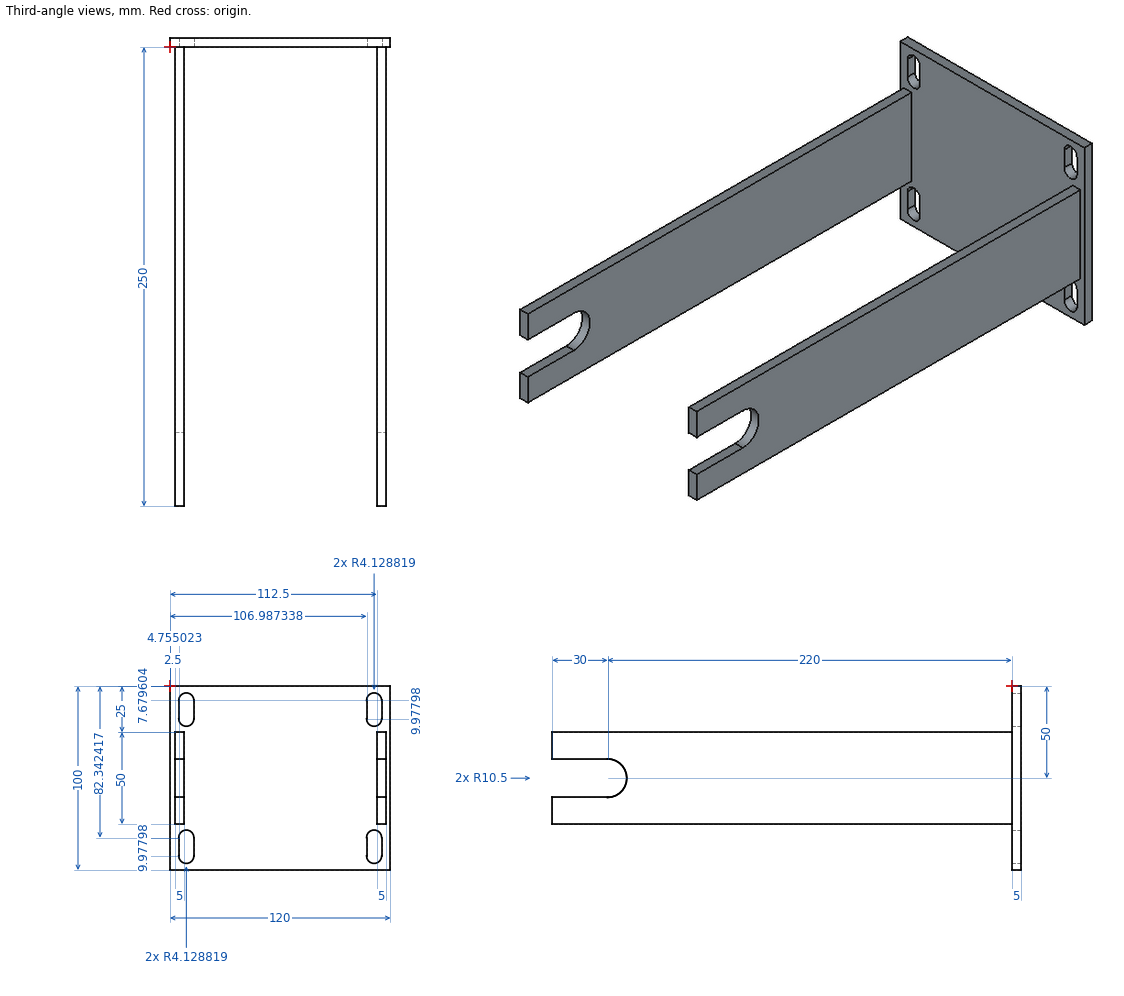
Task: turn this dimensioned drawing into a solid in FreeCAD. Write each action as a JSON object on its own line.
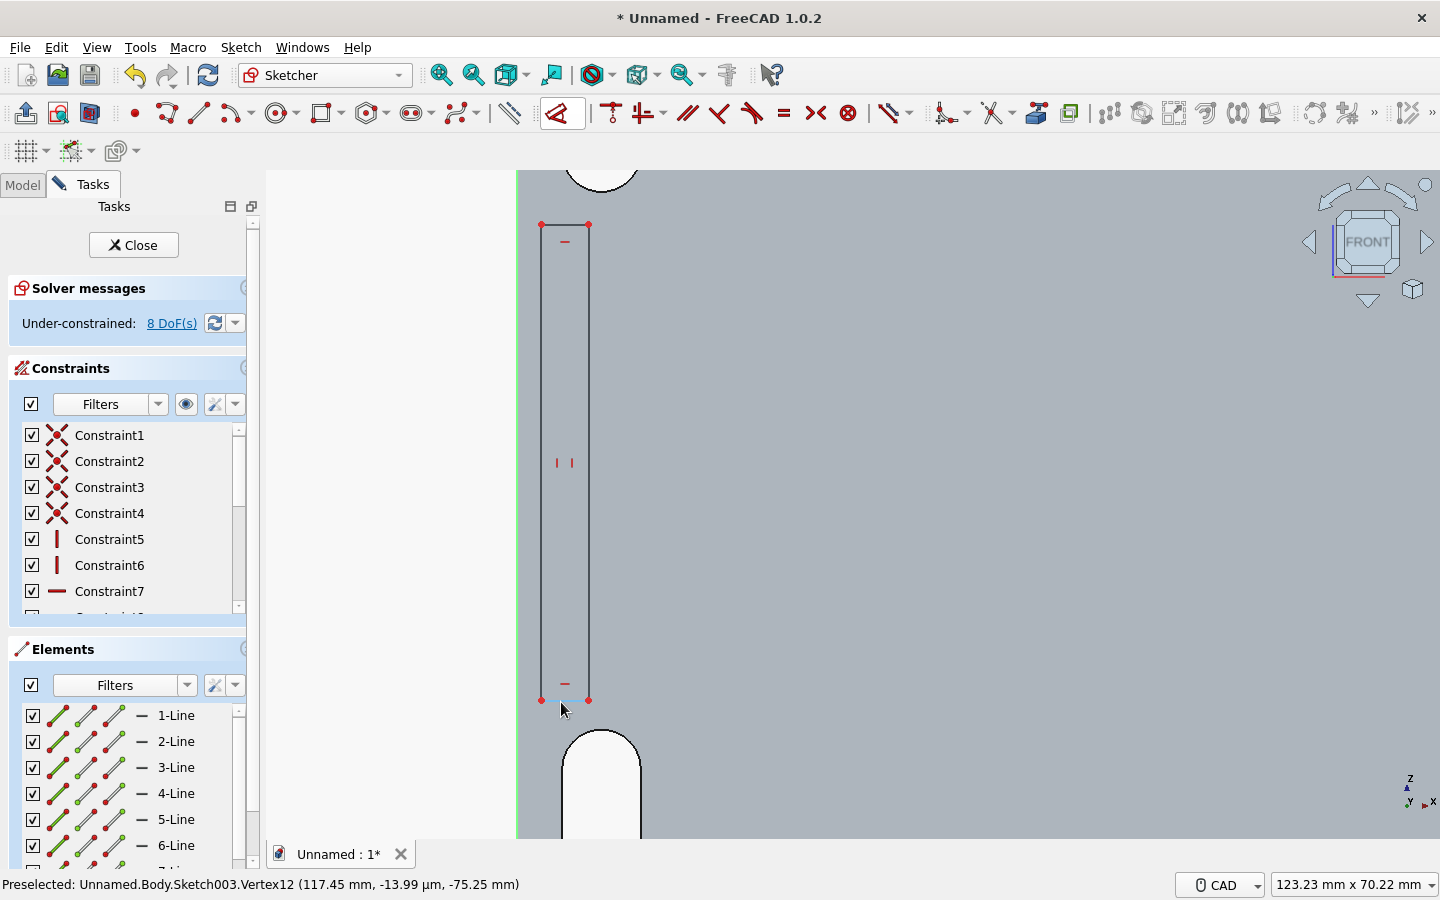
{"action": "left_click", "coordinate": [560, 701]}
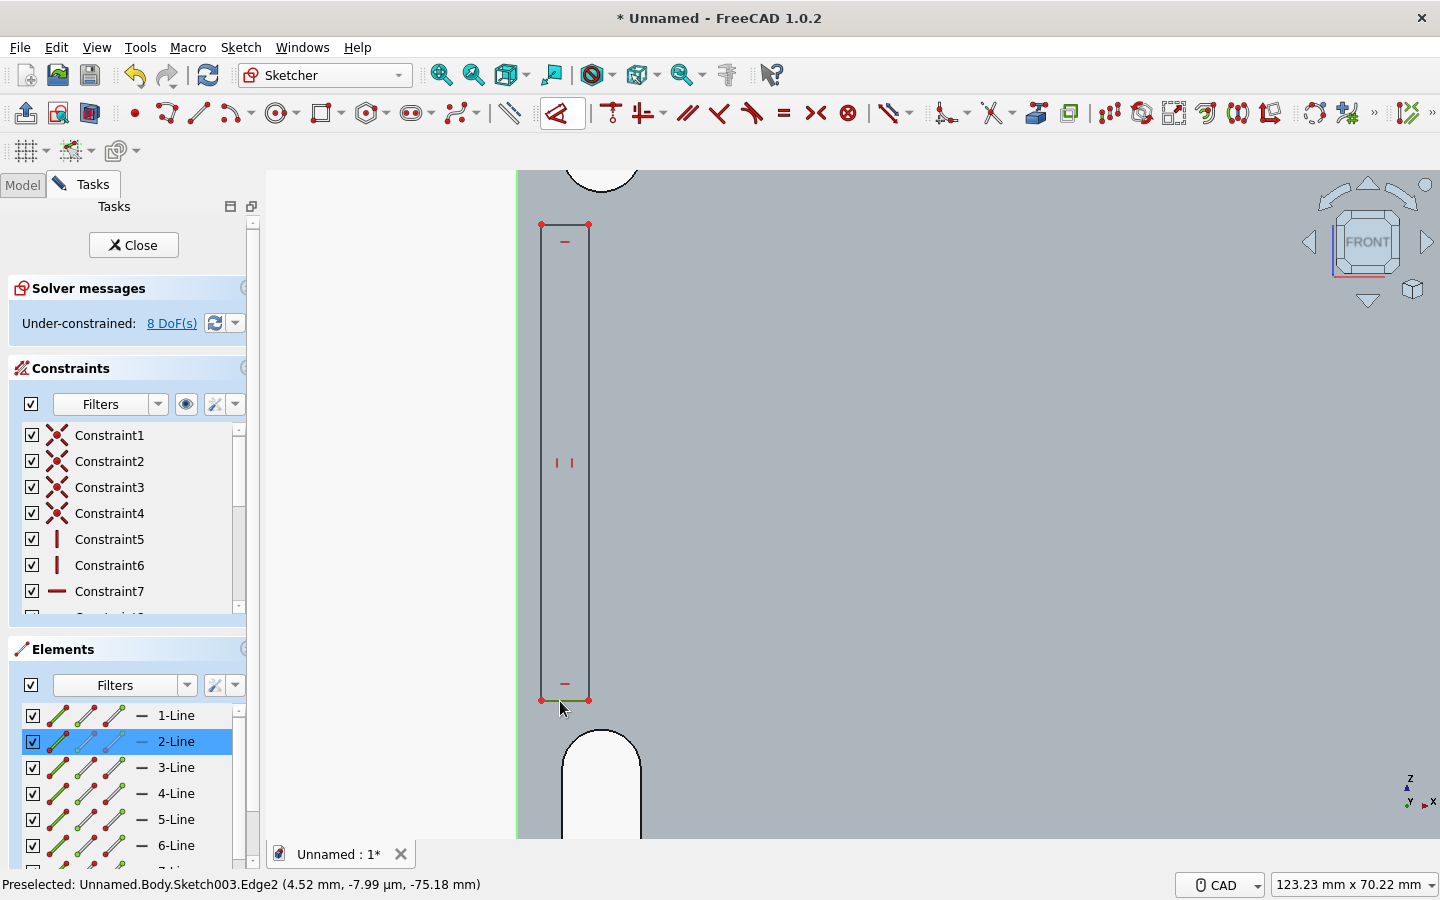
{"action": "key", "text": "l"}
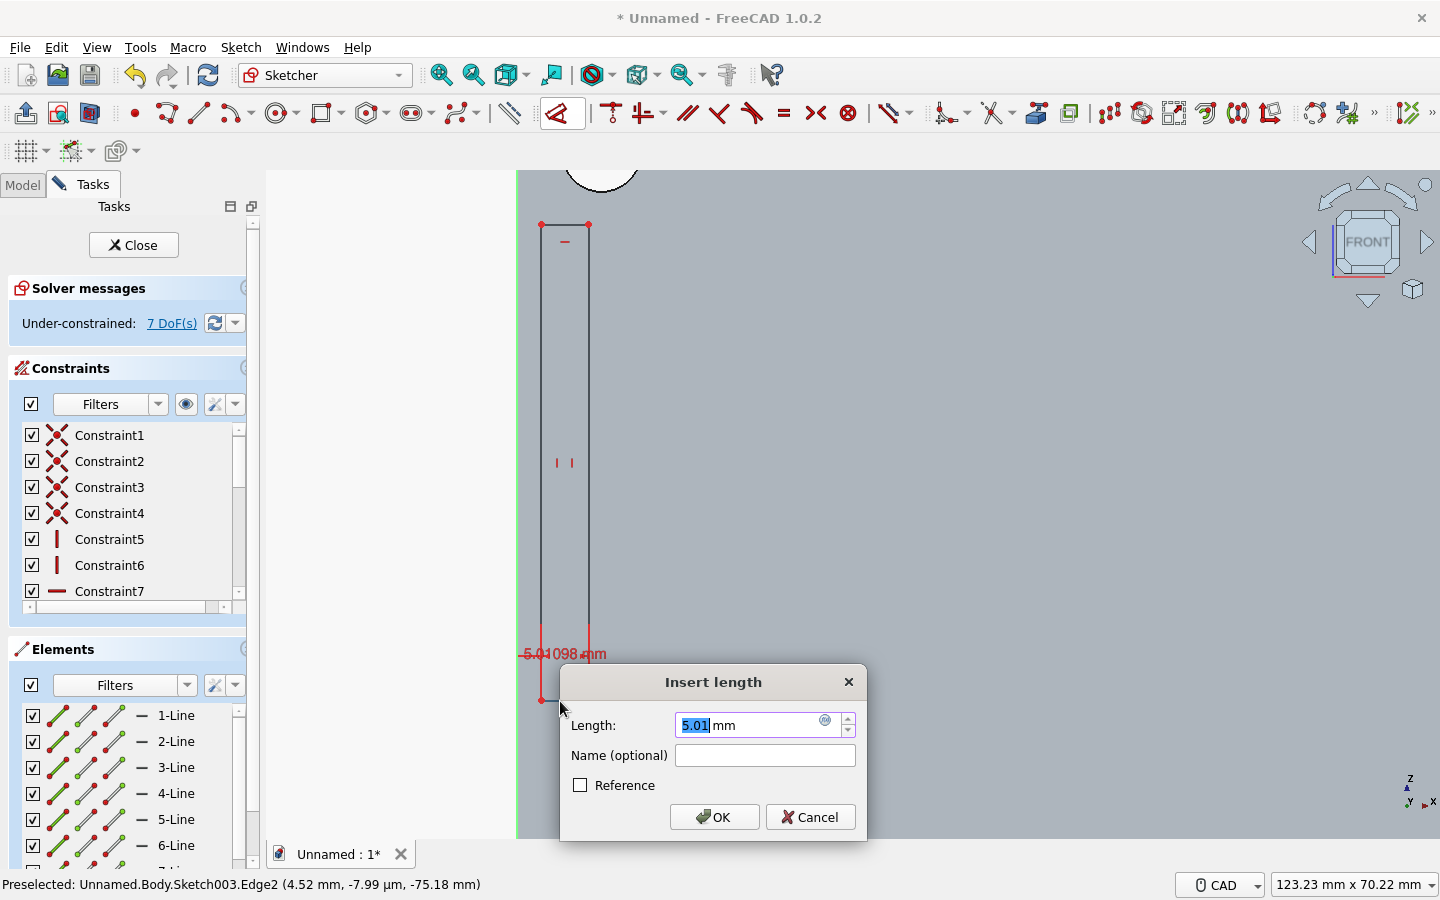
{"action": "type", "text": "5"}
{"action": "key", "text": "Return"}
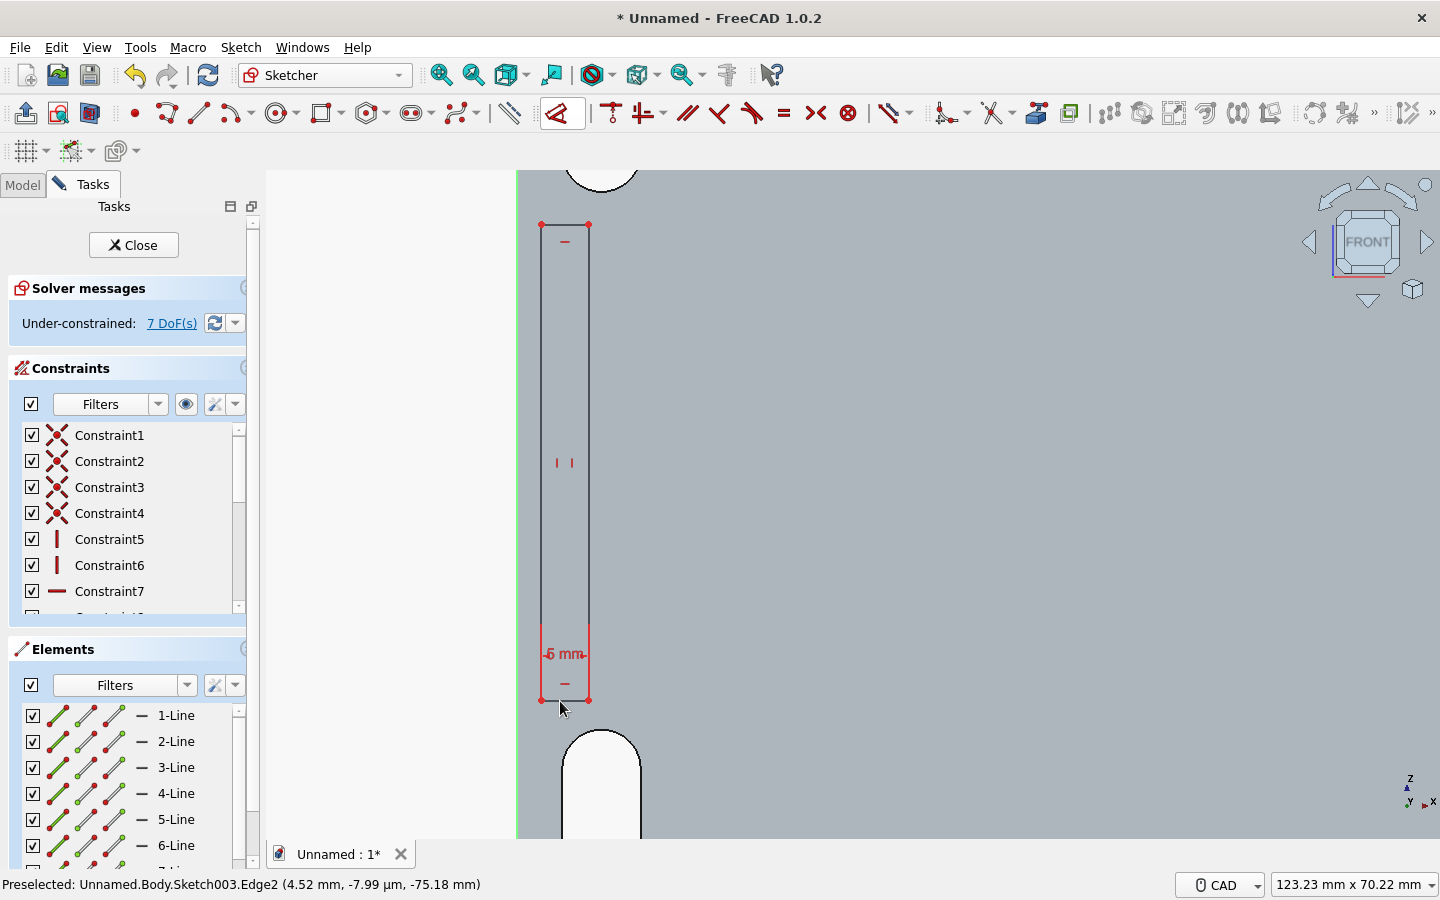
{"action": "scroll", "coordinate": [429, 703], "scroll_direction": "down", "scroll_amount": 3}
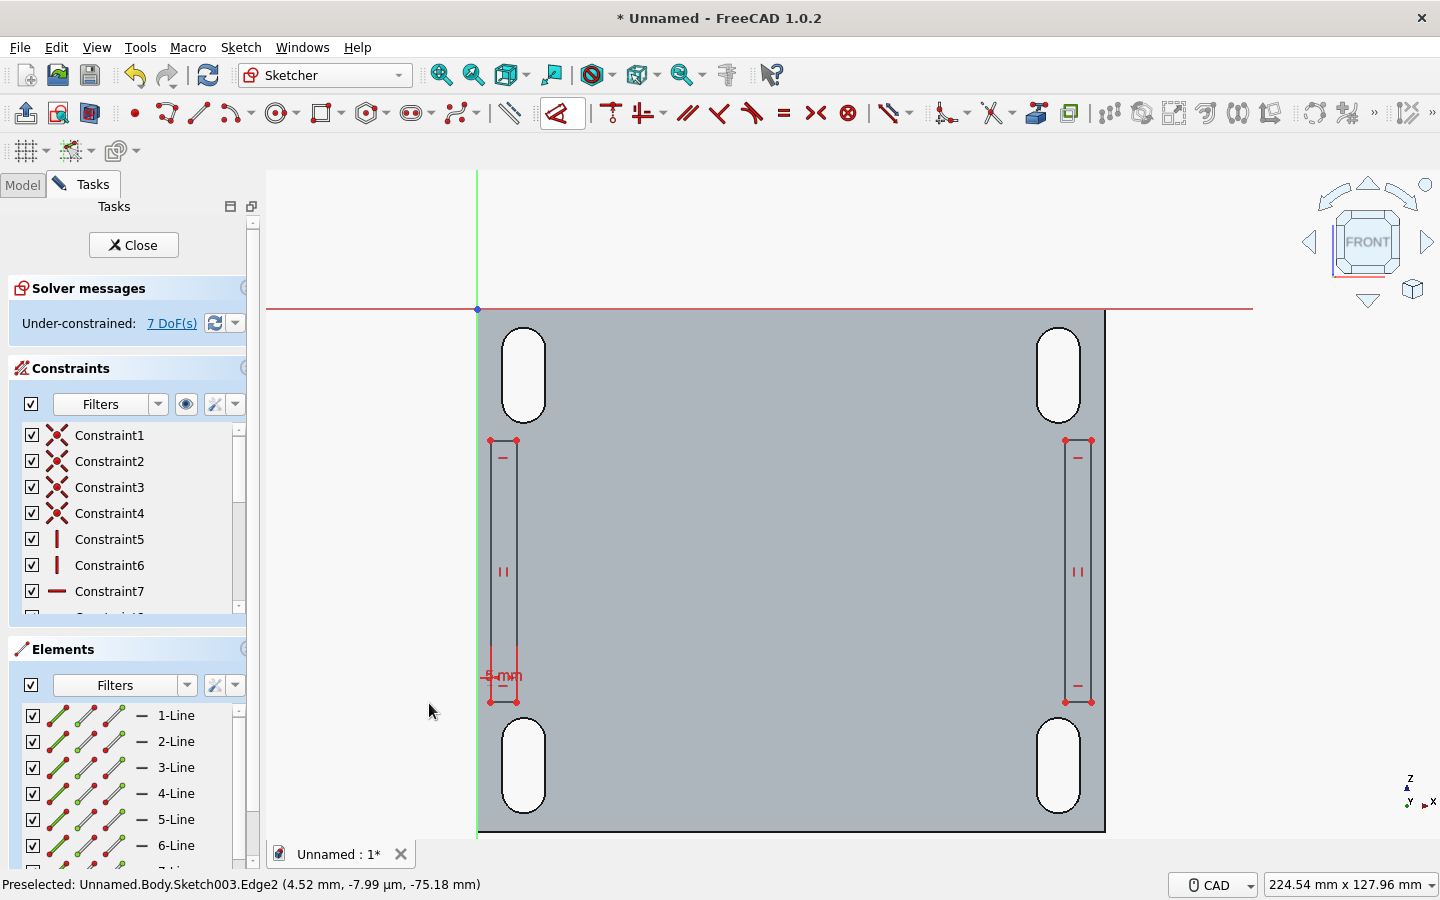
{"action": "scroll", "coordinate": [1073, 702], "scroll_direction": "up", "scroll_amount": 3}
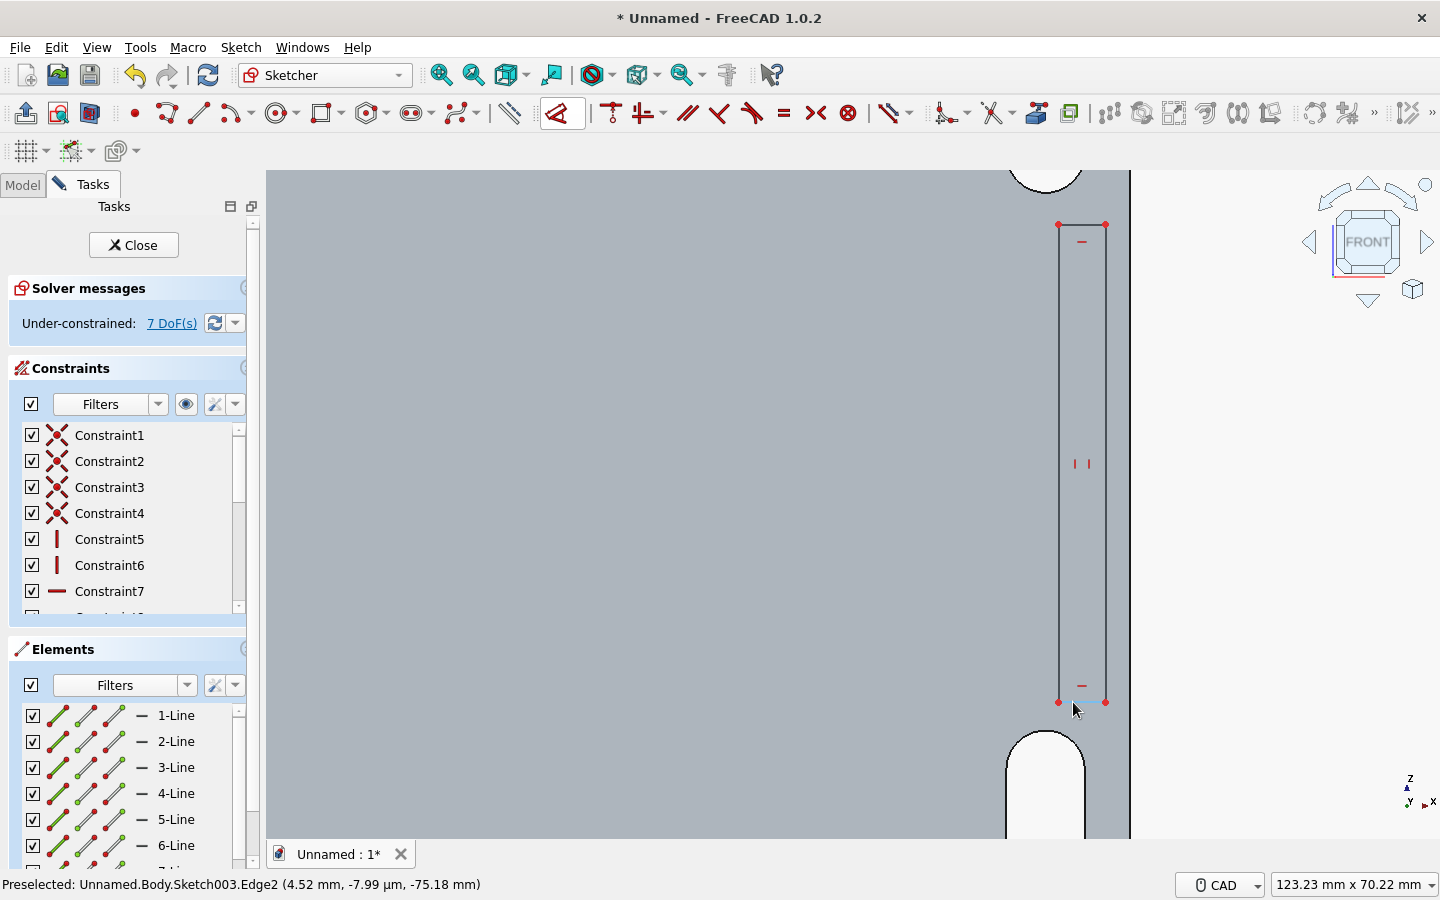
{"action": "left_click", "coordinate": [1073, 702]}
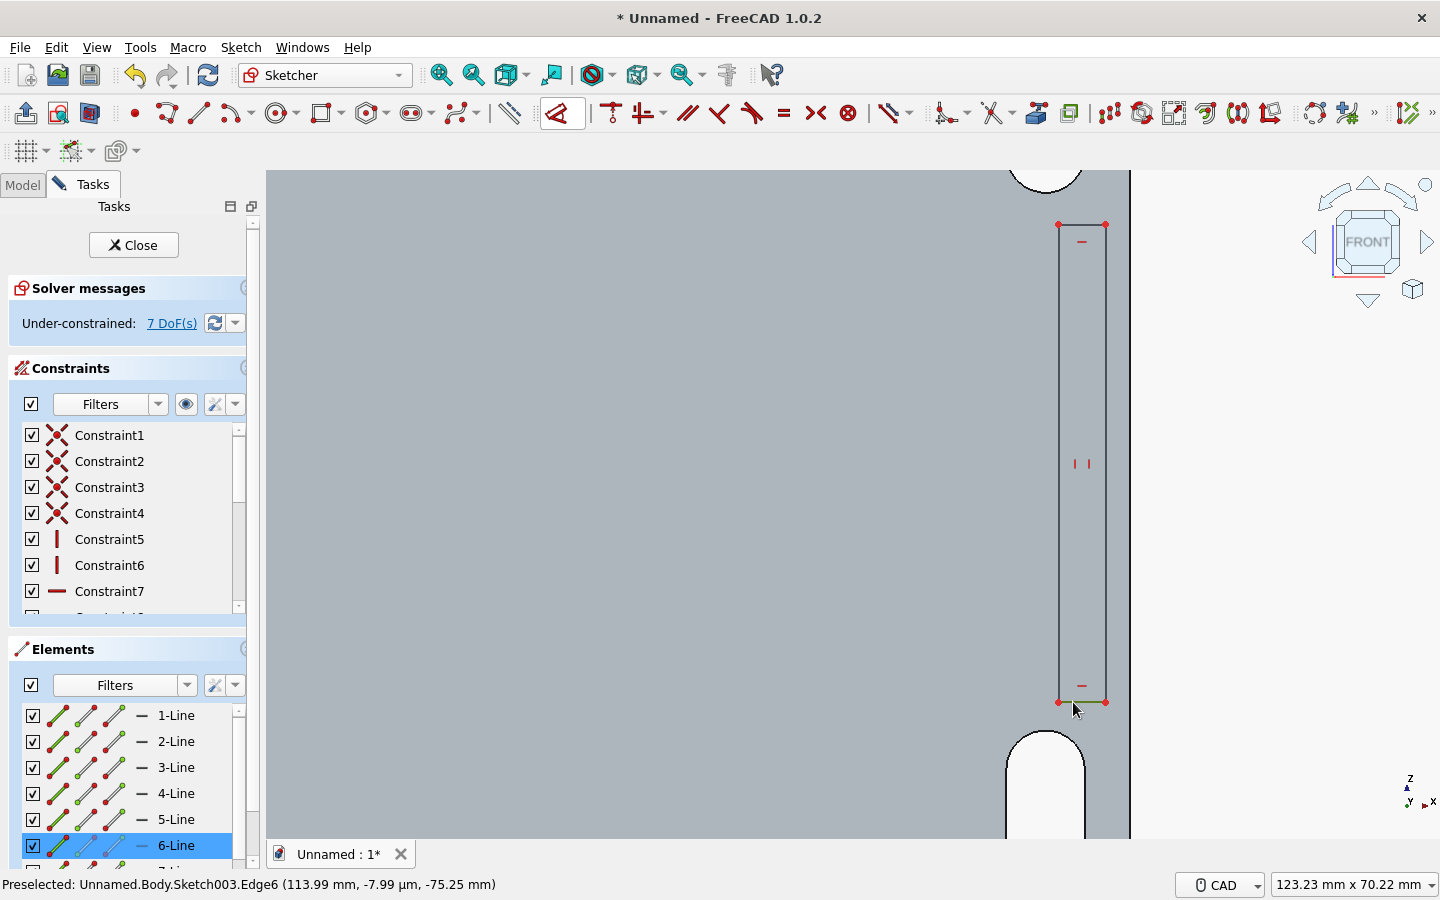
{"action": "left_click", "coordinate": [580, 114]}